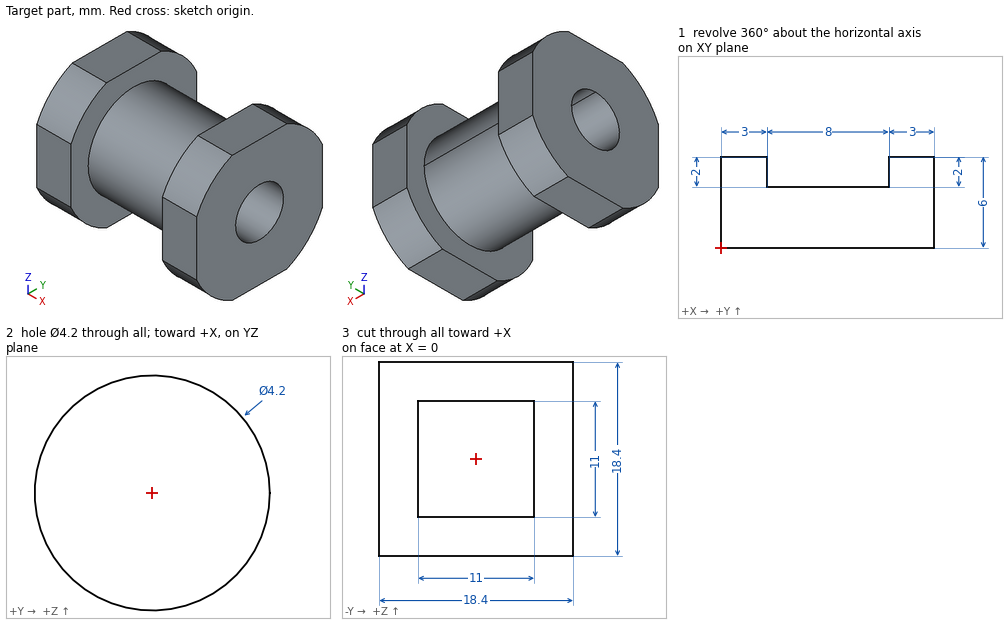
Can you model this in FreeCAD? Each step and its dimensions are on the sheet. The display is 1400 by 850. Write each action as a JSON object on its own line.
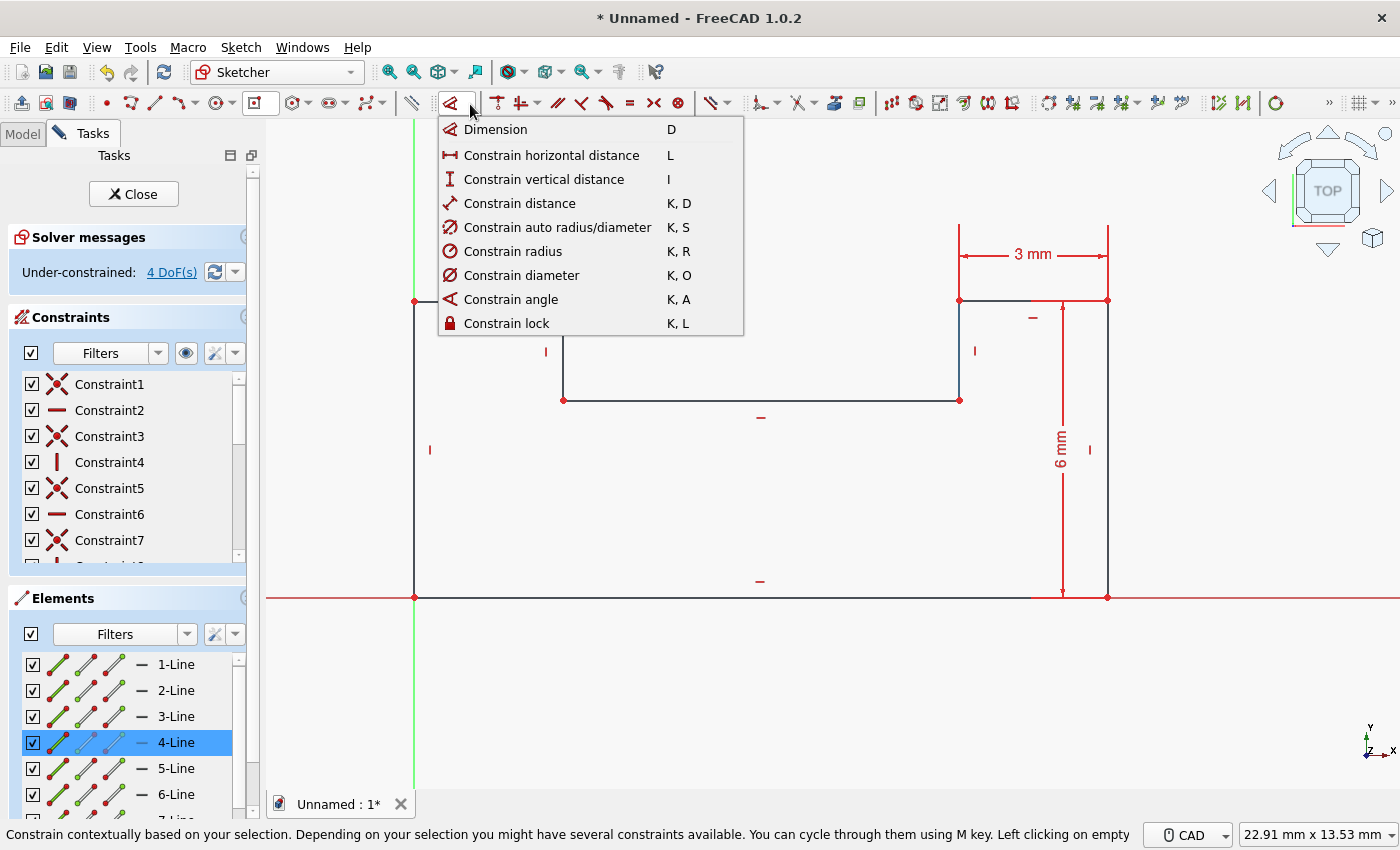
{"action": "left_click", "coordinate": [591, 179]}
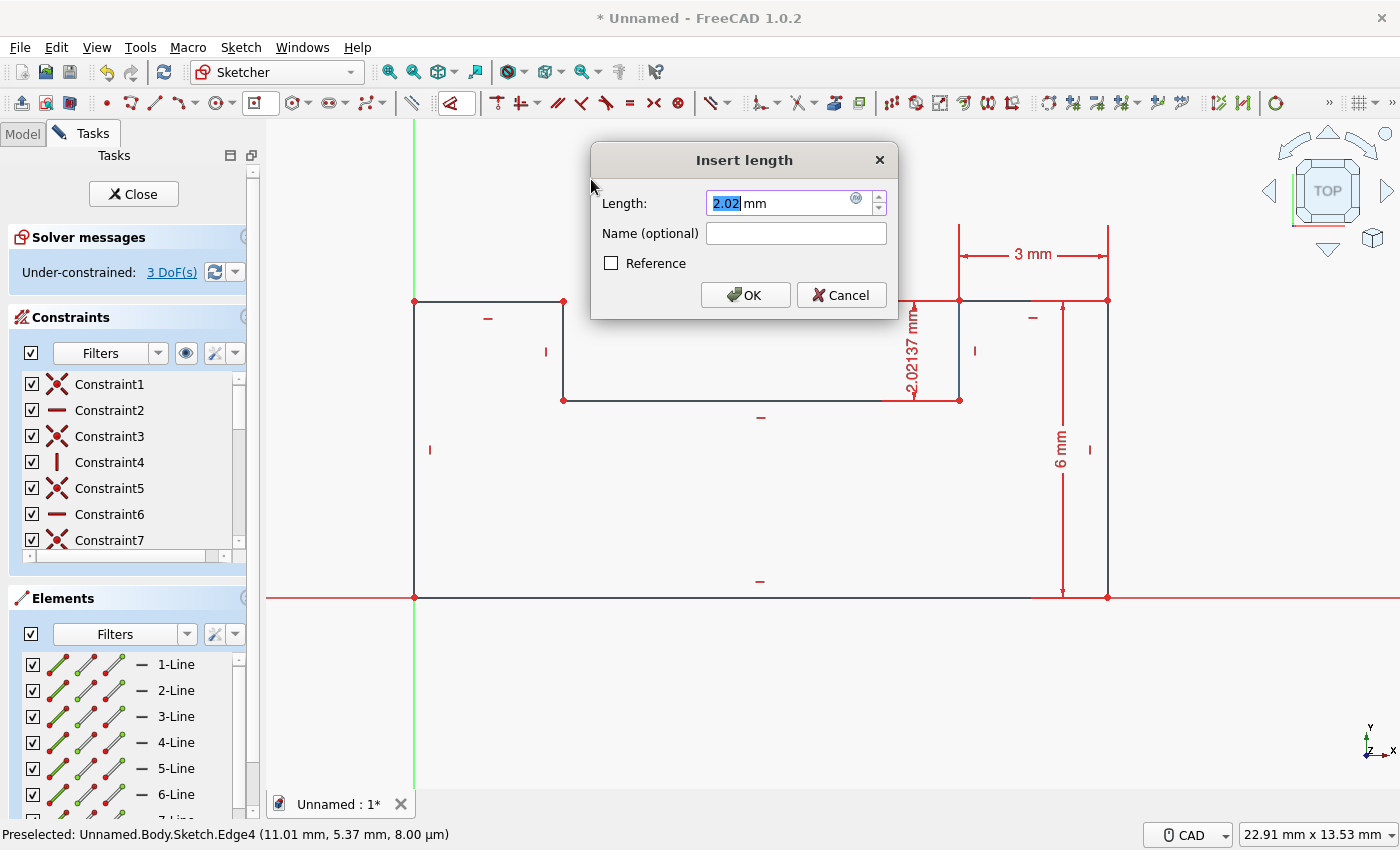
{"action": "type", "text": "2"}
{"action": "key", "text": "Return"}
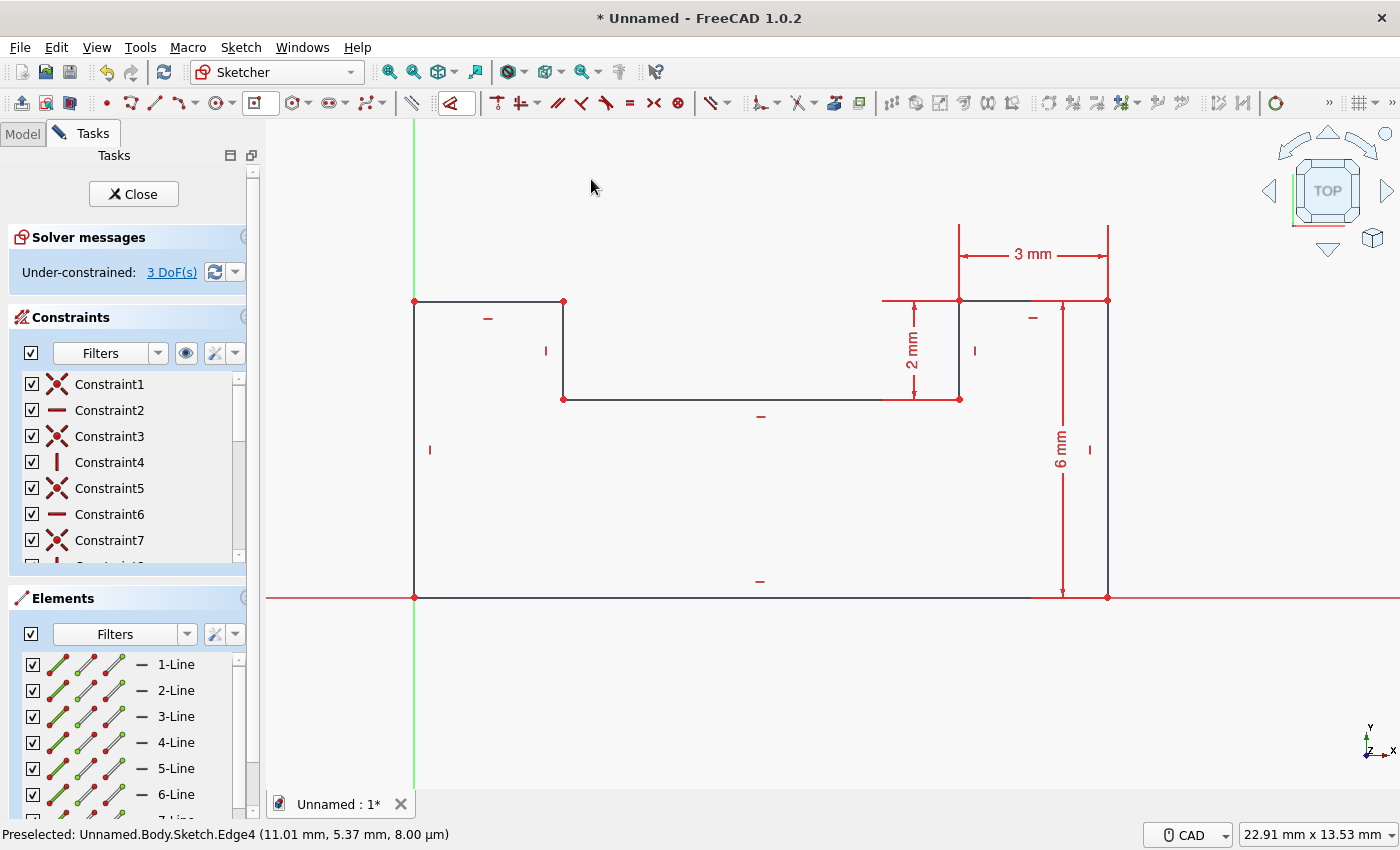
{"action": "left_click", "coordinate": [840, 400]}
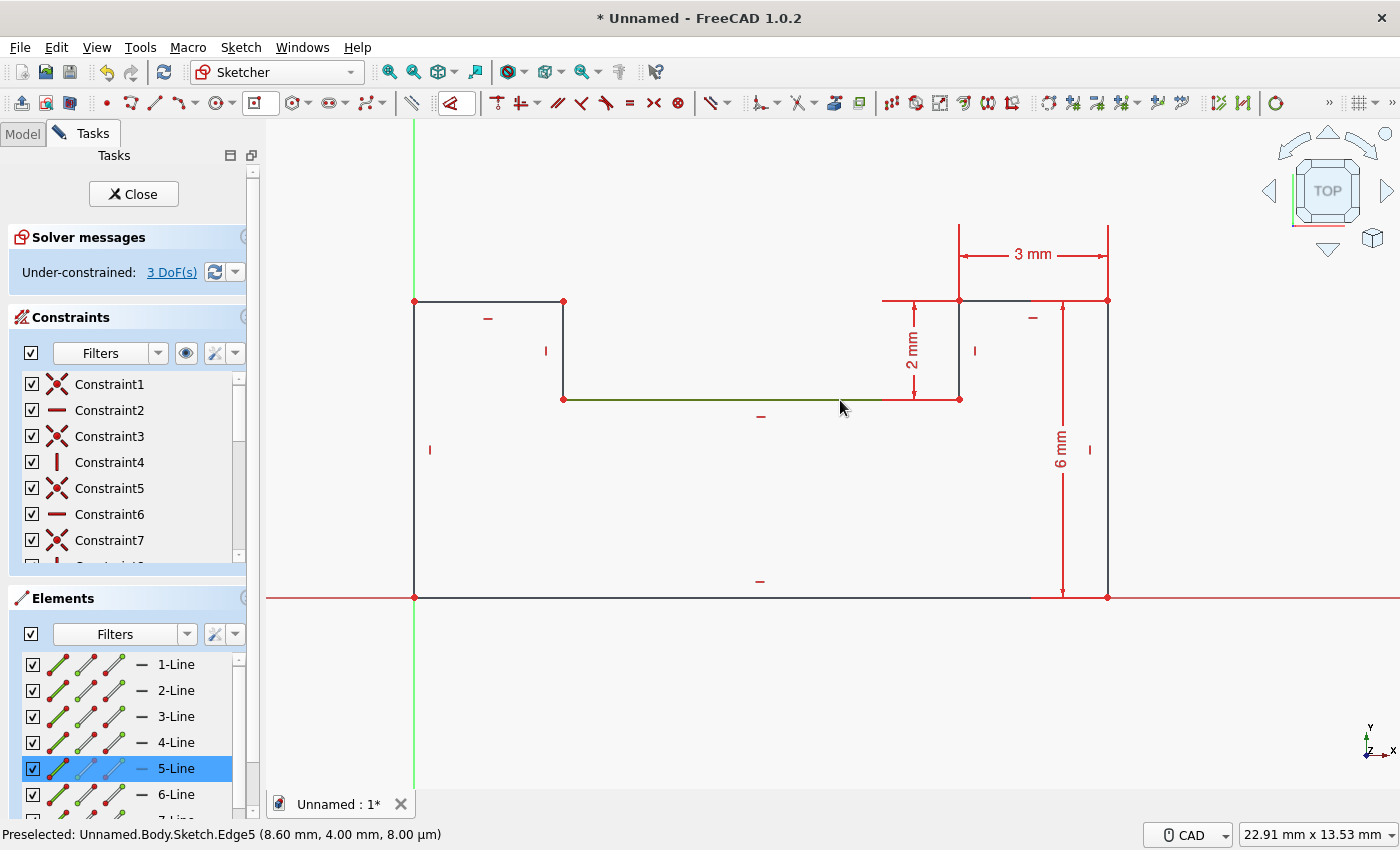
{"action": "left_click", "coordinate": [470, 104]}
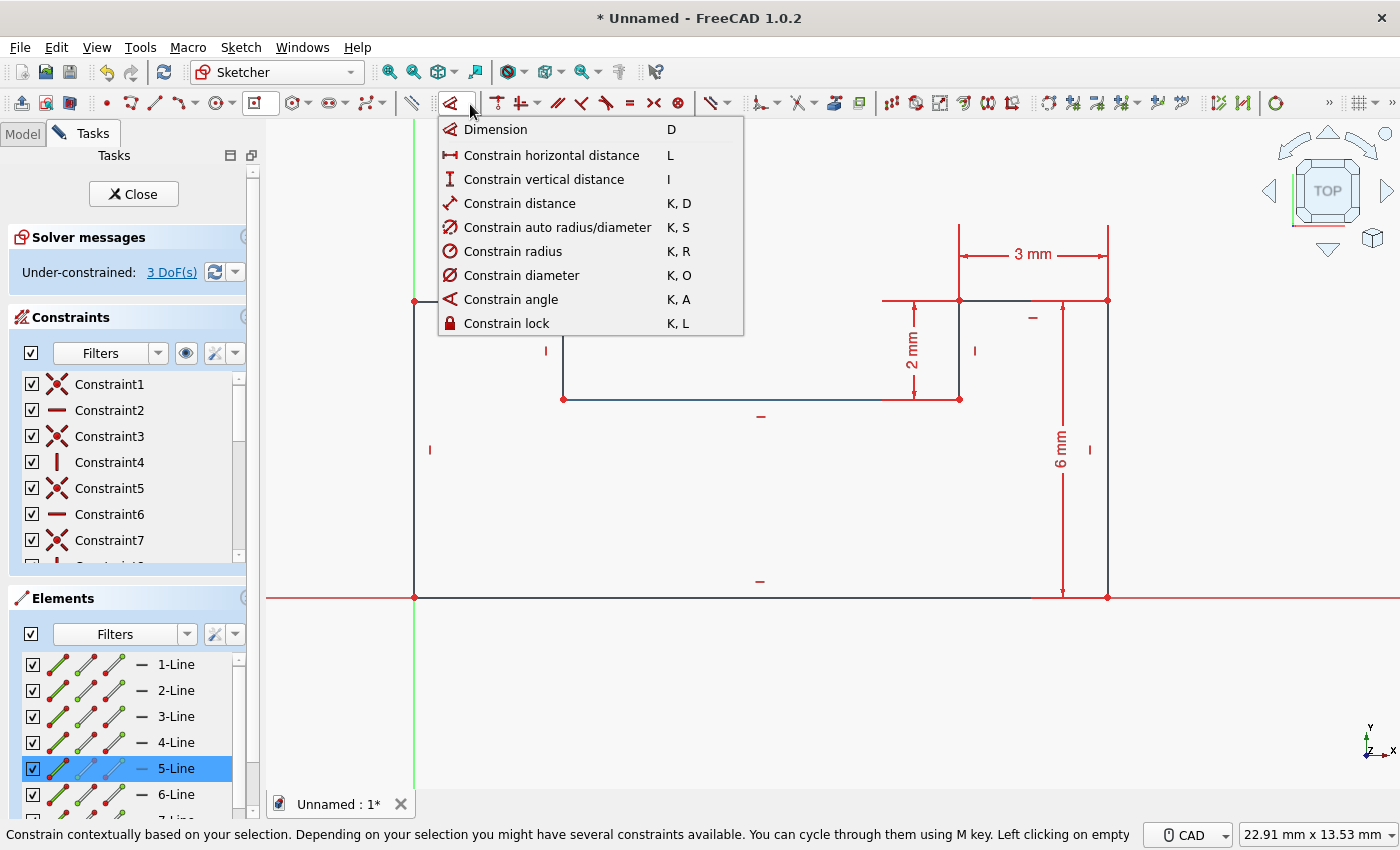
{"action": "left_click", "coordinate": [591, 155]}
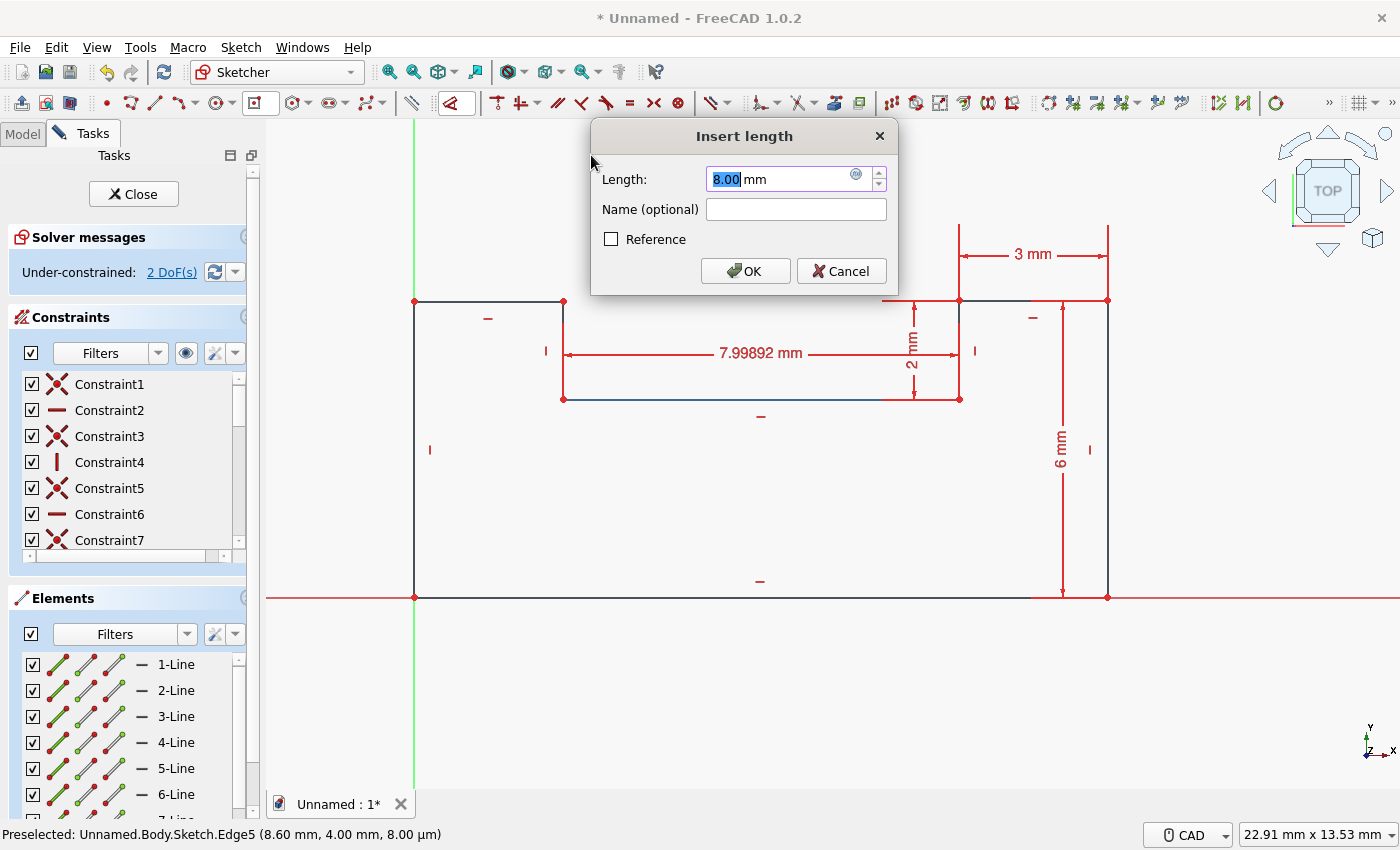
{"action": "type", "text": "8"}
{"action": "key", "text": "Return"}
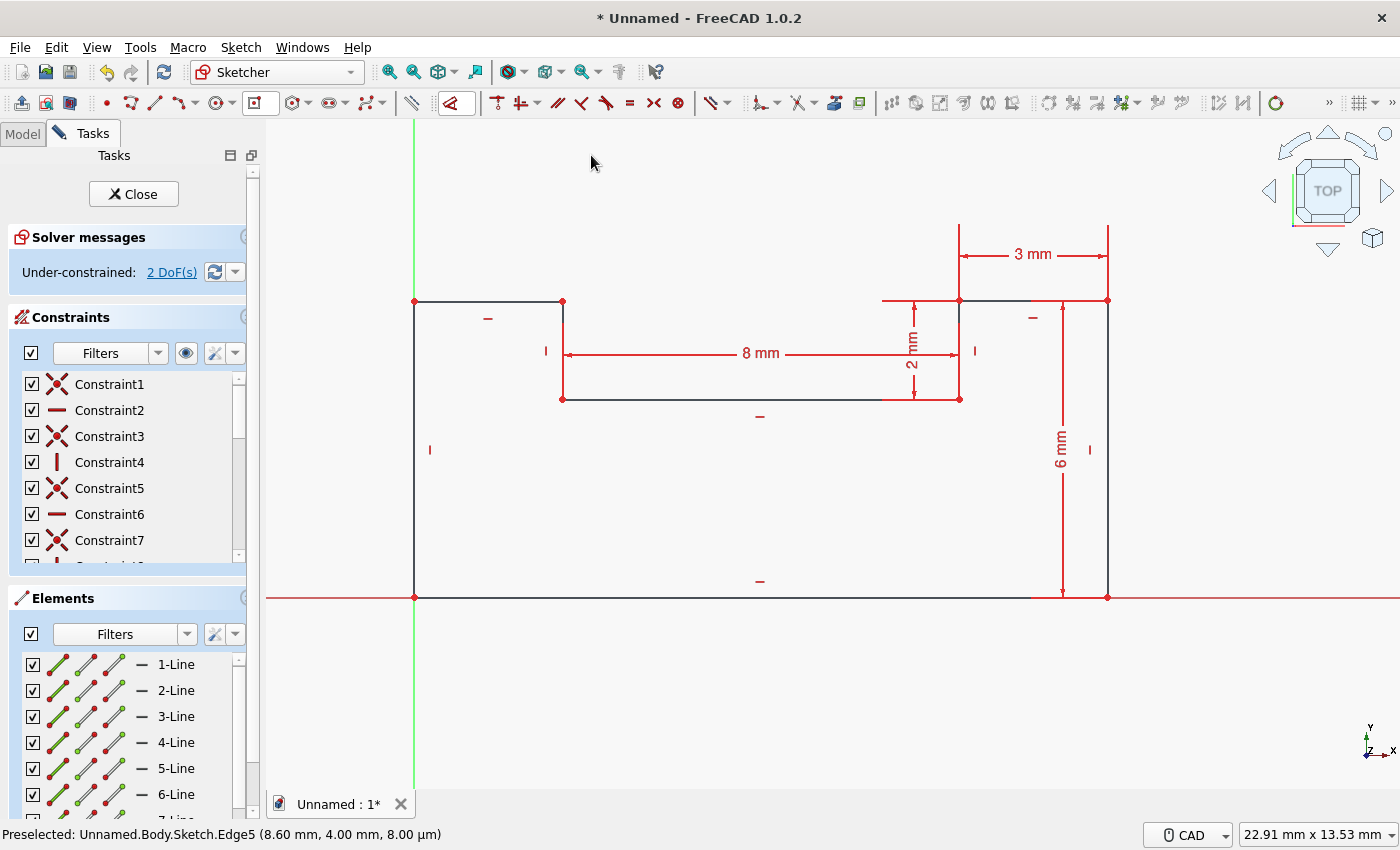
{"action": "left_click", "coordinate": [563, 371]}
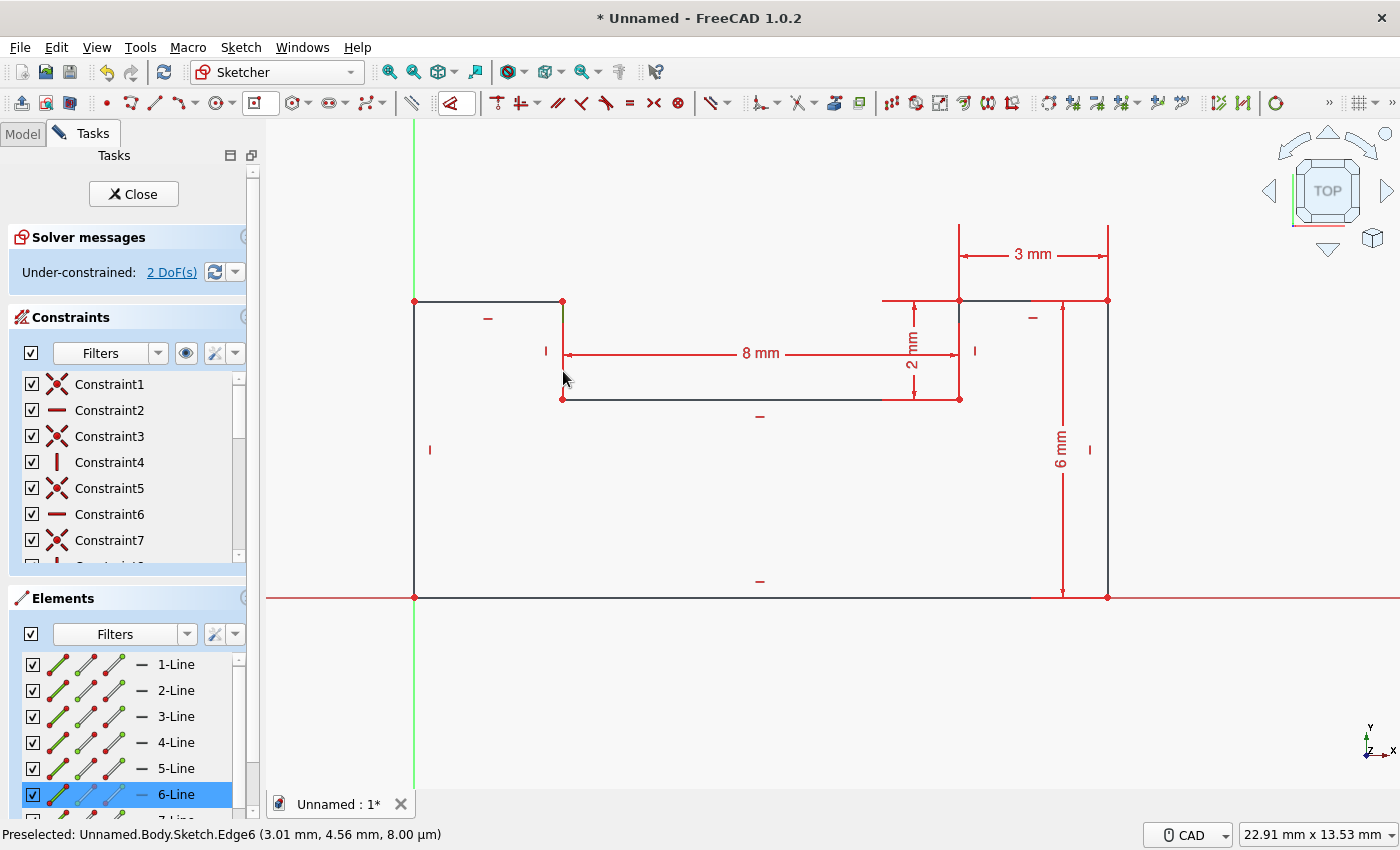
{"action": "left_click", "coordinate": [470, 104]}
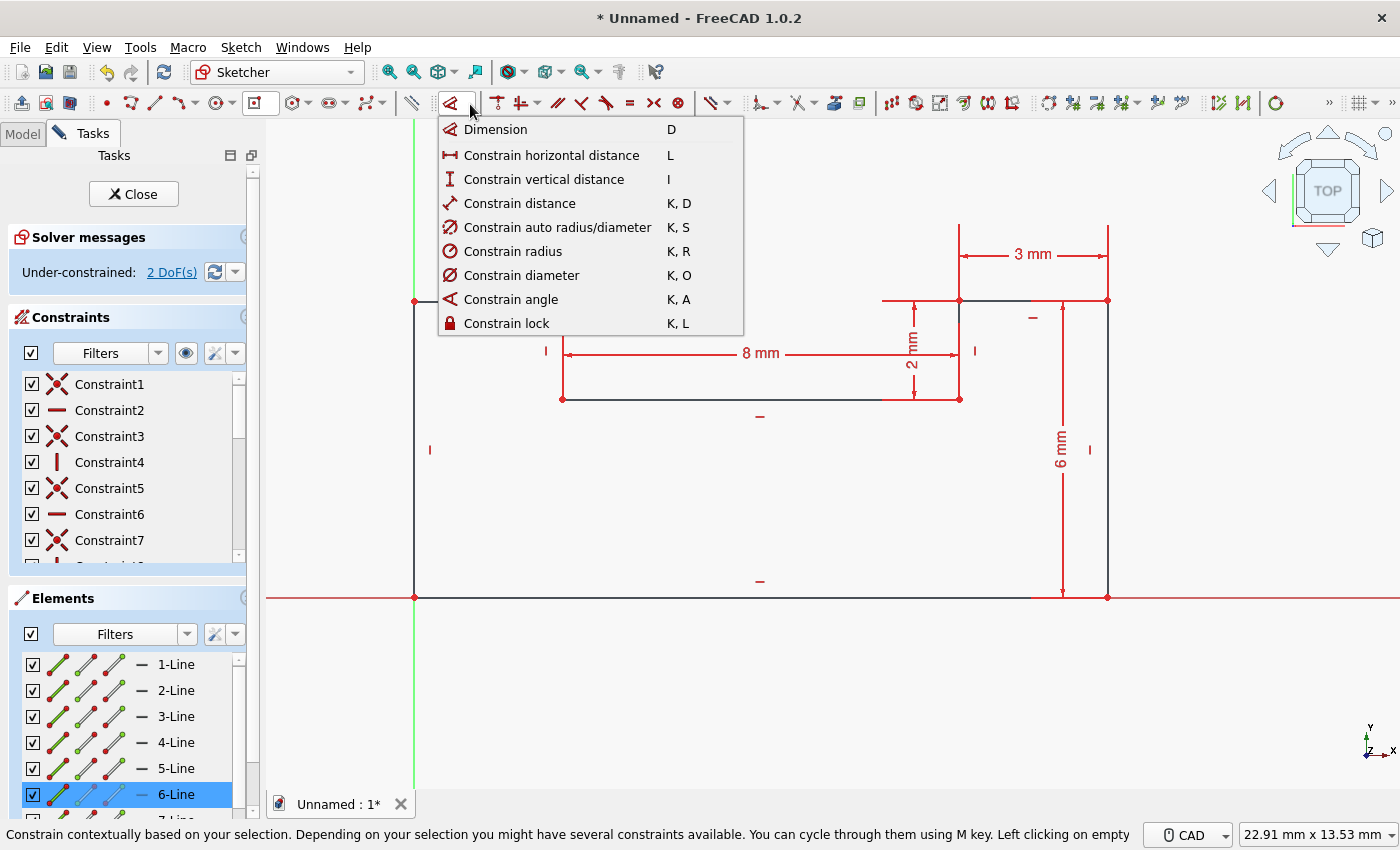
{"action": "left_click", "coordinate": [591, 179]}